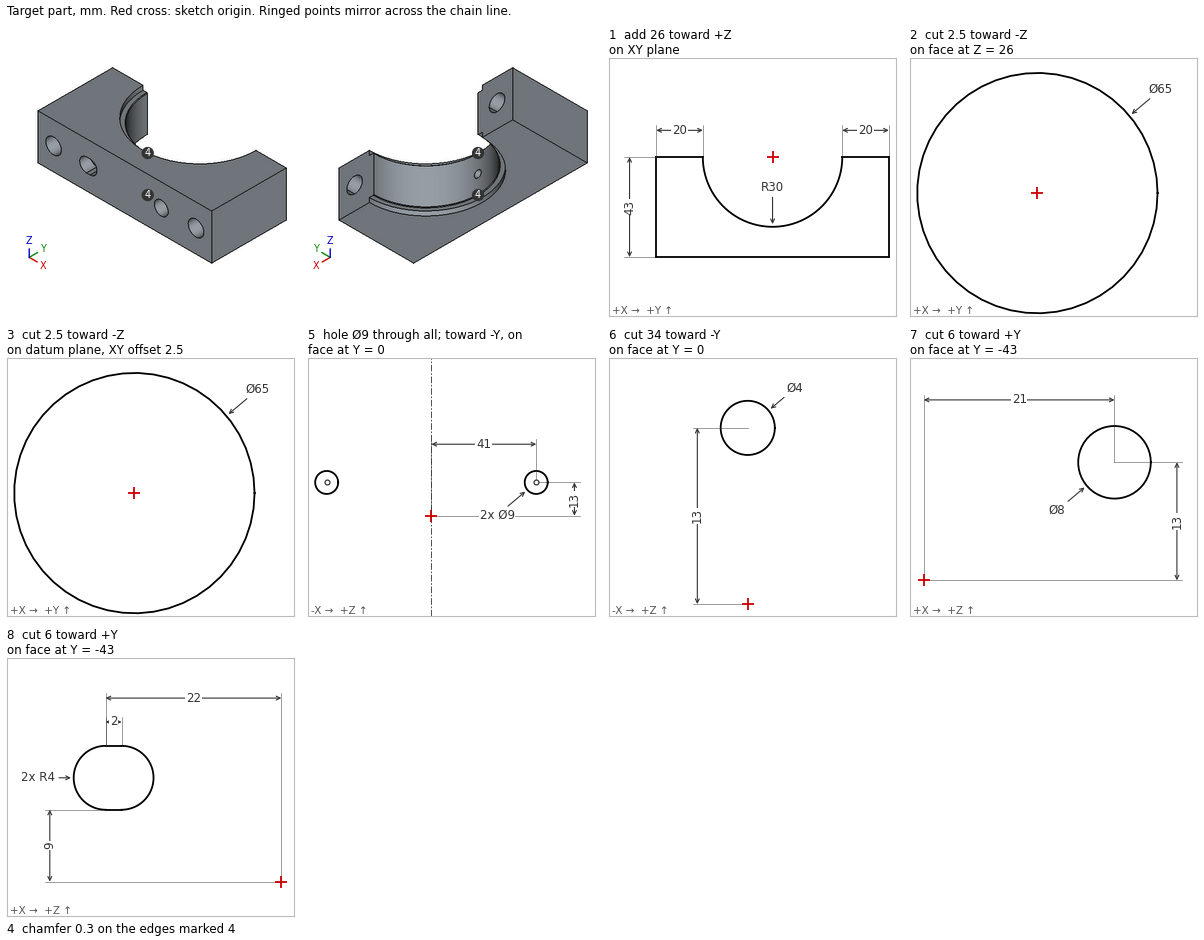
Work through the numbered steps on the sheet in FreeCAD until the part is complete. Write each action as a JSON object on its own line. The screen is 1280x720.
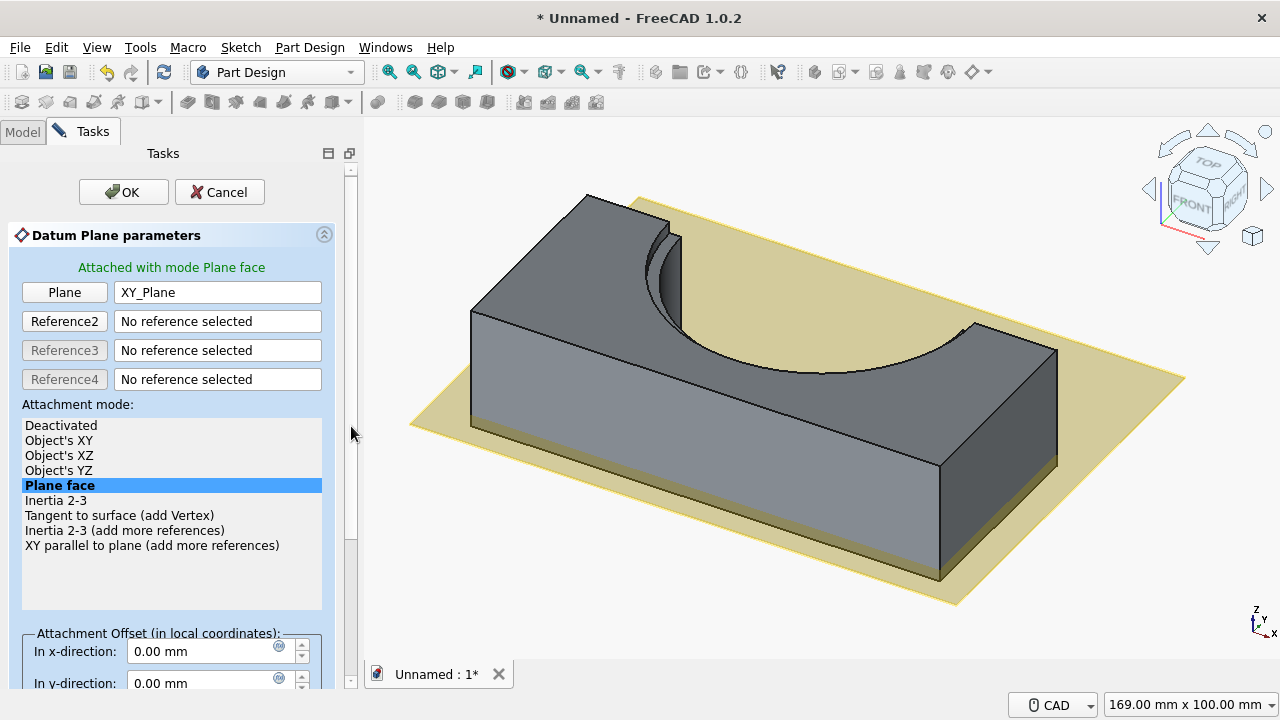
{"action": "left_click", "coordinate": [124, 192]}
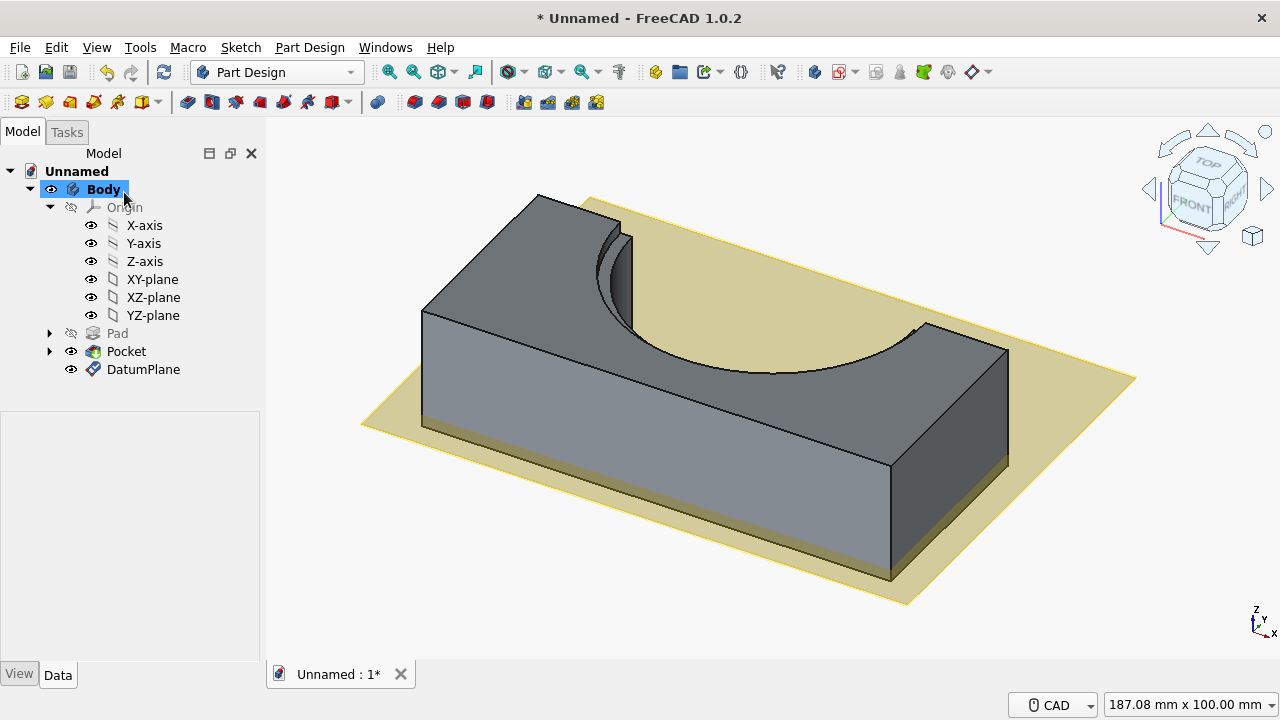
{"action": "left_click", "coordinate": [116, 369]}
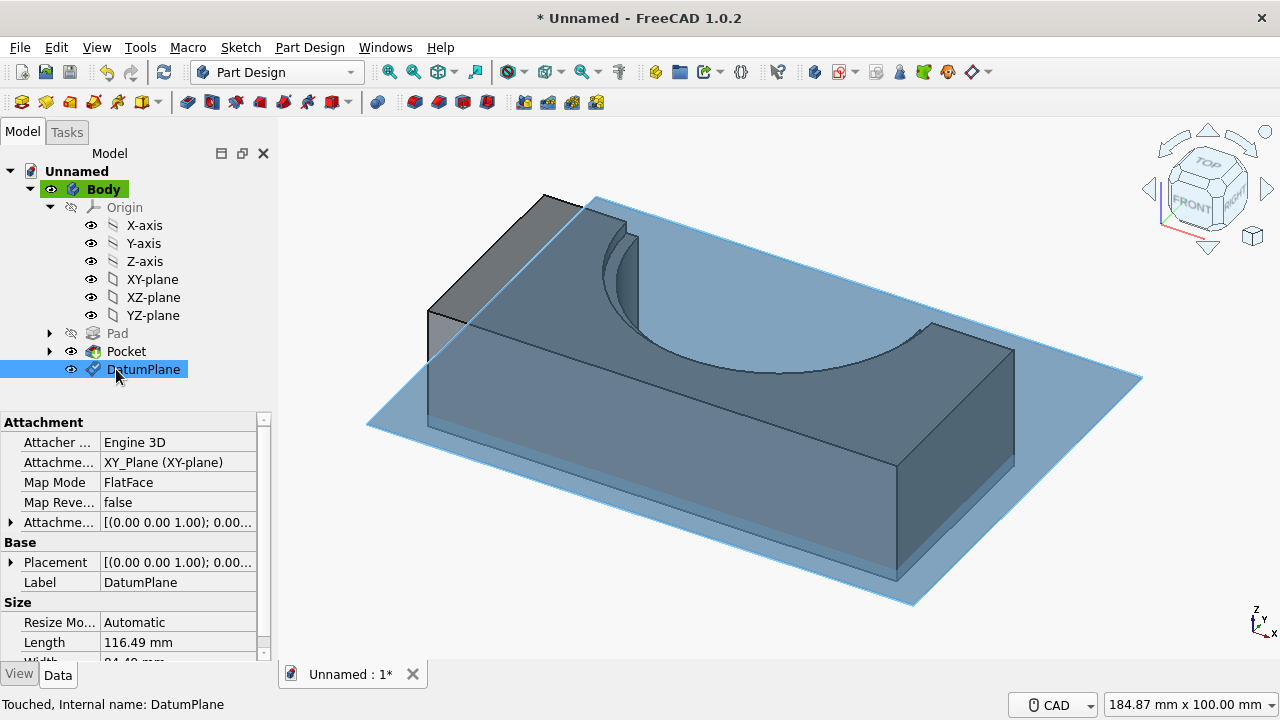
{"action": "left_click", "coordinate": [840, 72]}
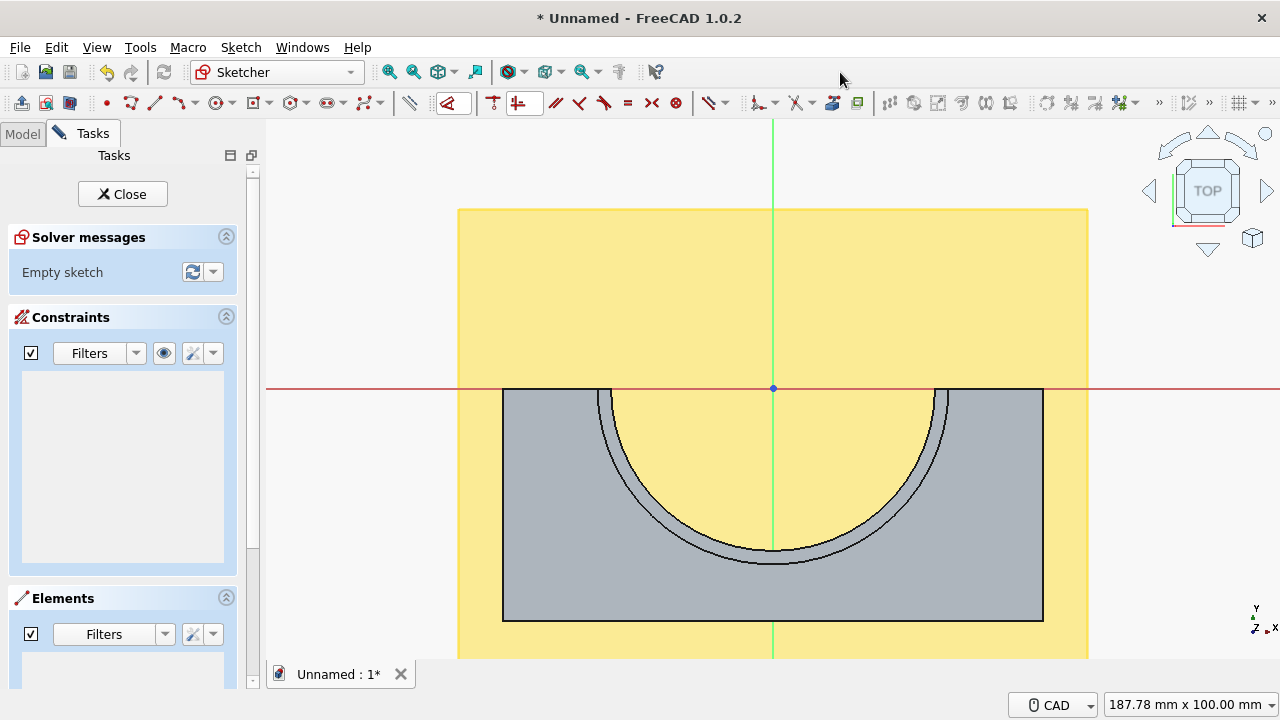
{"action": "left_click", "coordinate": [70, 104]}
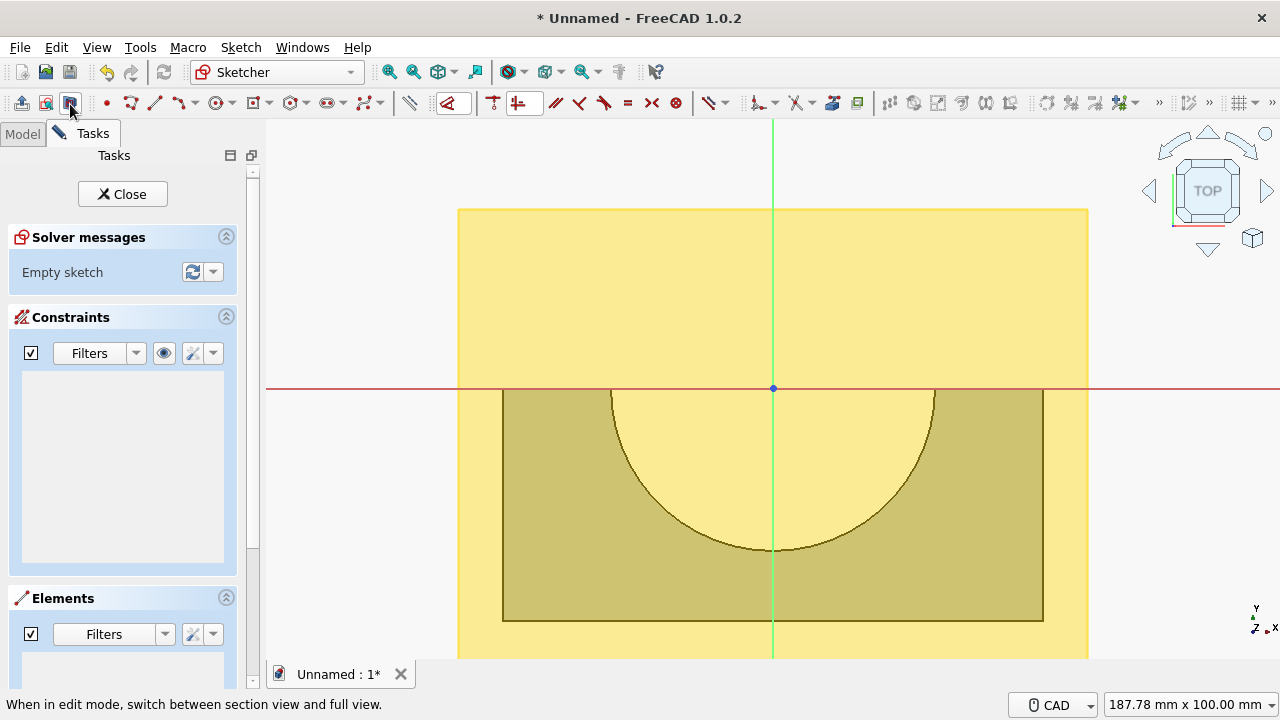
{"action": "left_click", "coordinate": [216, 104]}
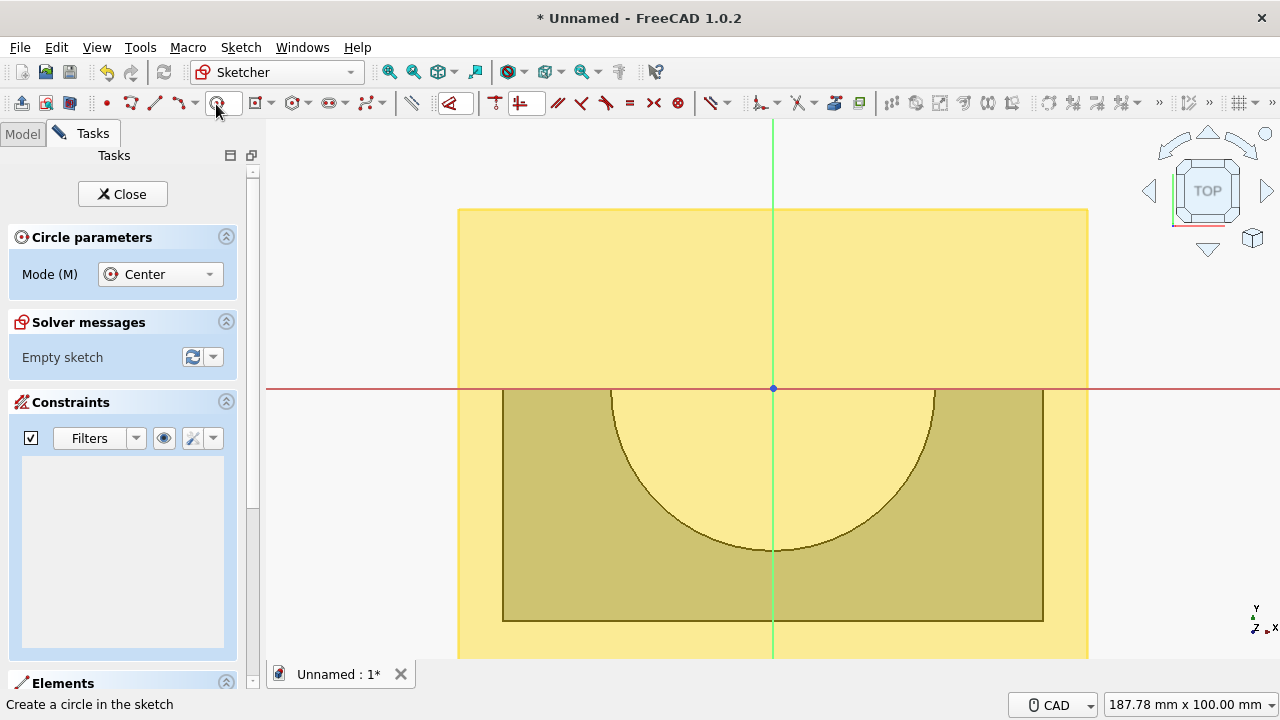
{"action": "left_click", "coordinate": [773, 389]}
{"action": "left_click", "coordinate": [897, 265]}
{"action": "key", "text": "Escape"}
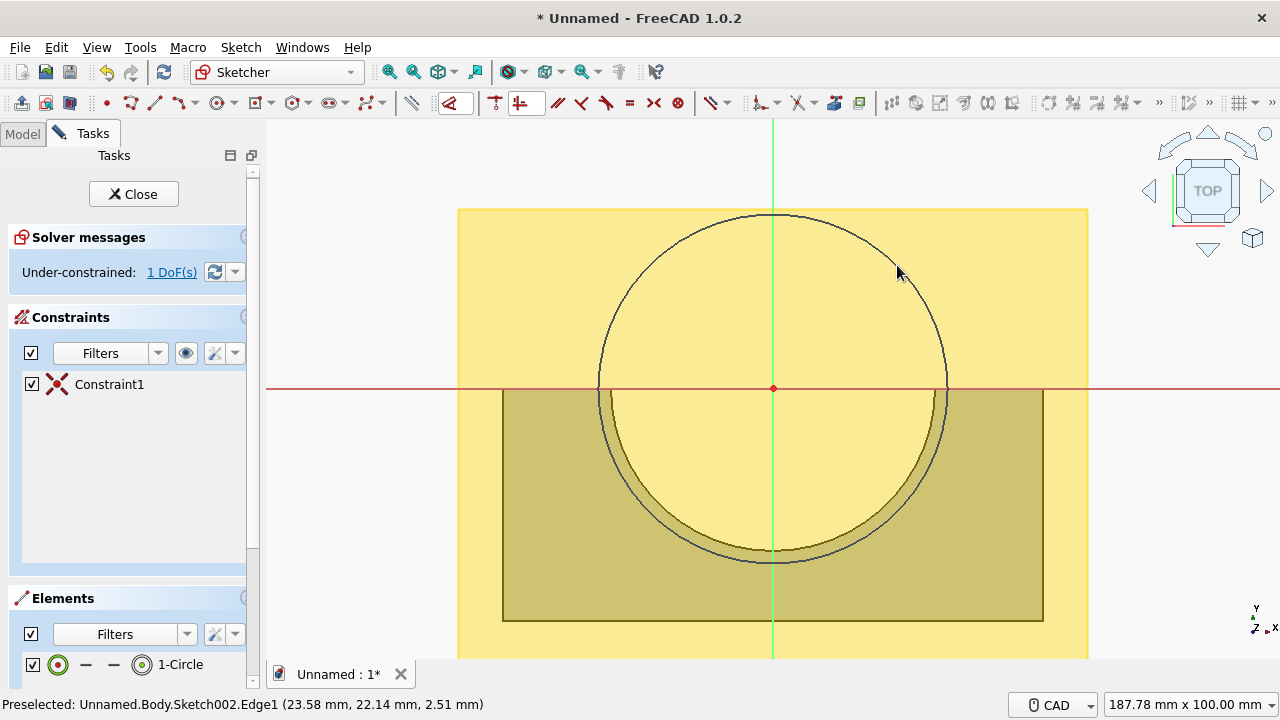
{"action": "left_click", "coordinate": [896, 265]}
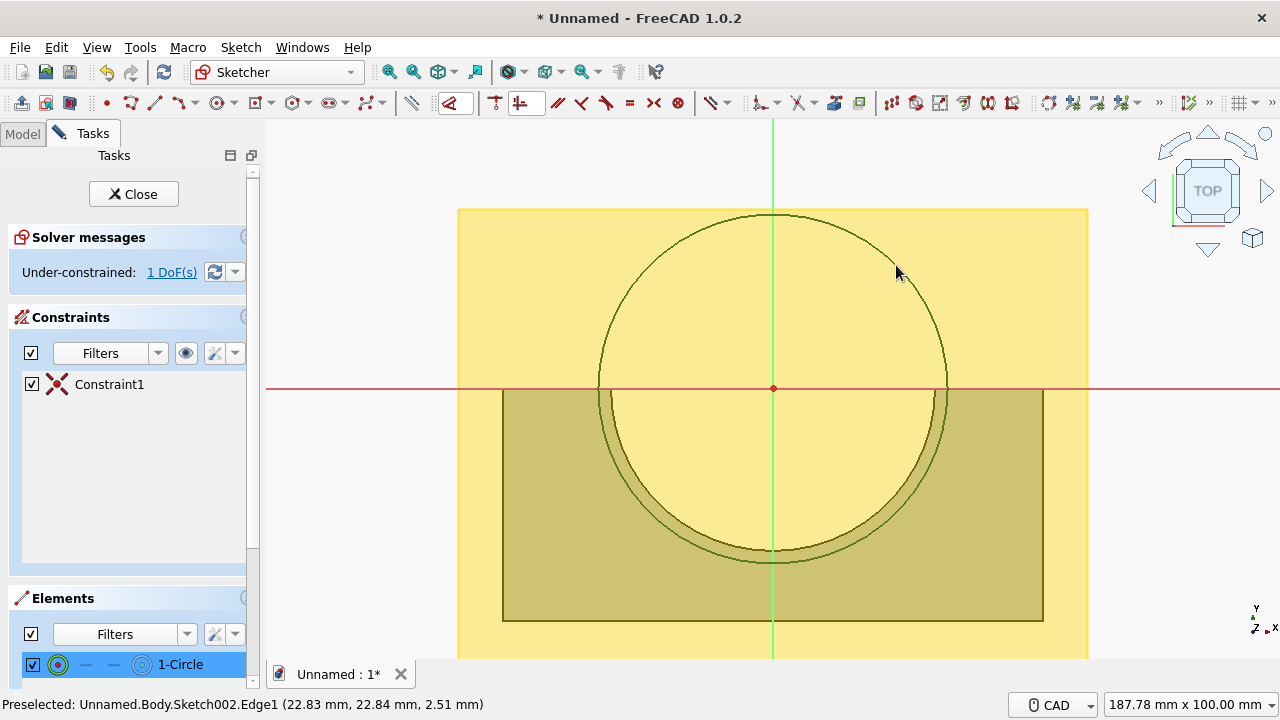
{"action": "left_click", "coordinate": [468, 104]}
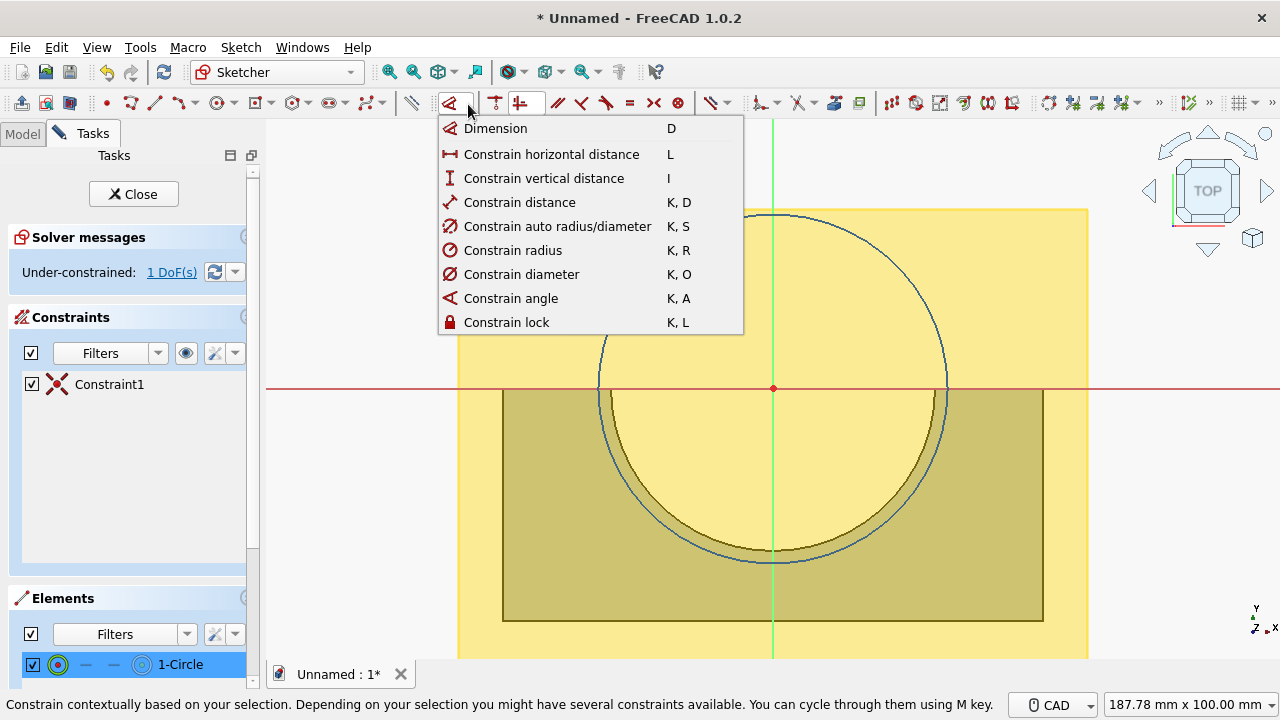
{"action": "left_click", "coordinate": [591, 274]}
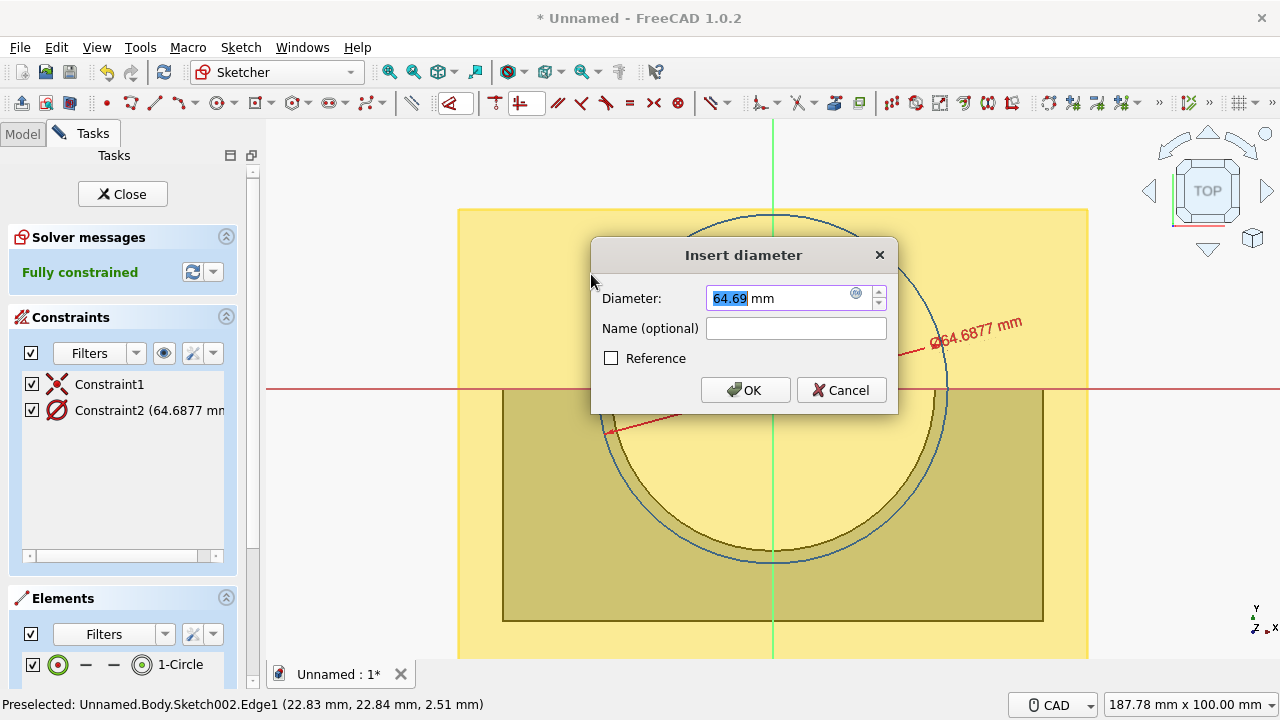
{"action": "type", "text": "65"}
{"action": "key", "text": "Return"}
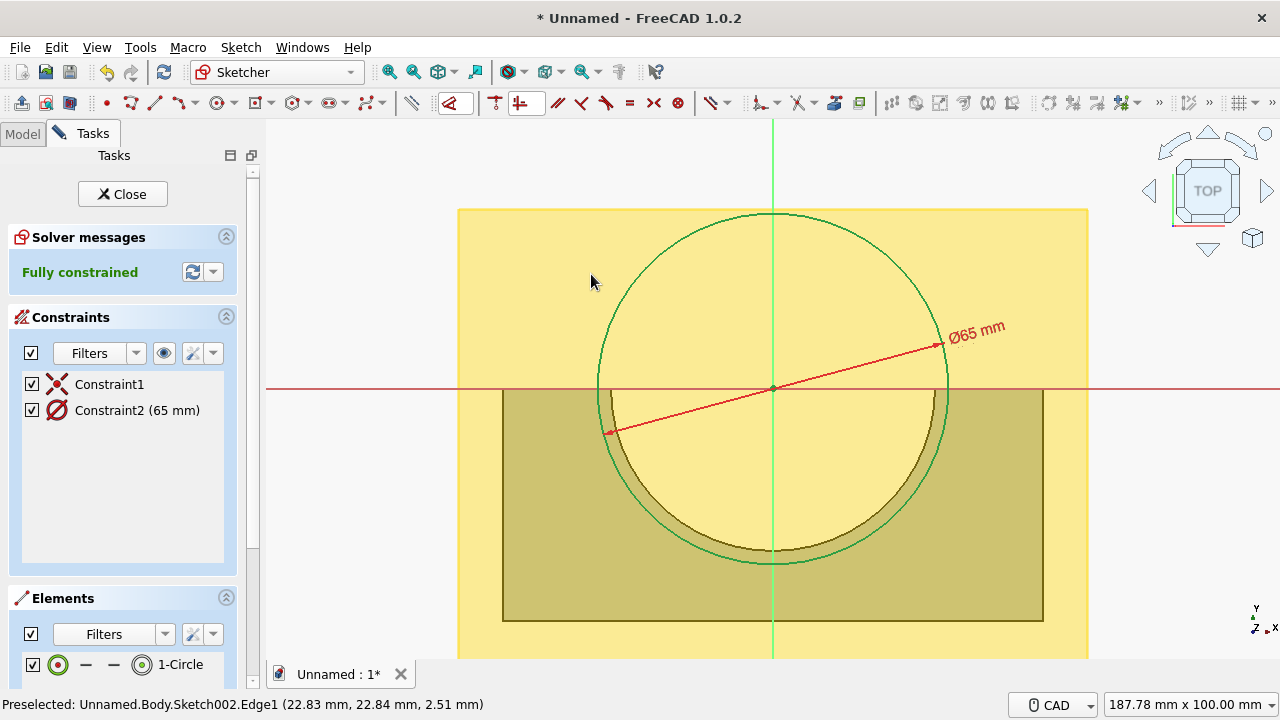
{"action": "left_click", "coordinate": [123, 194]}